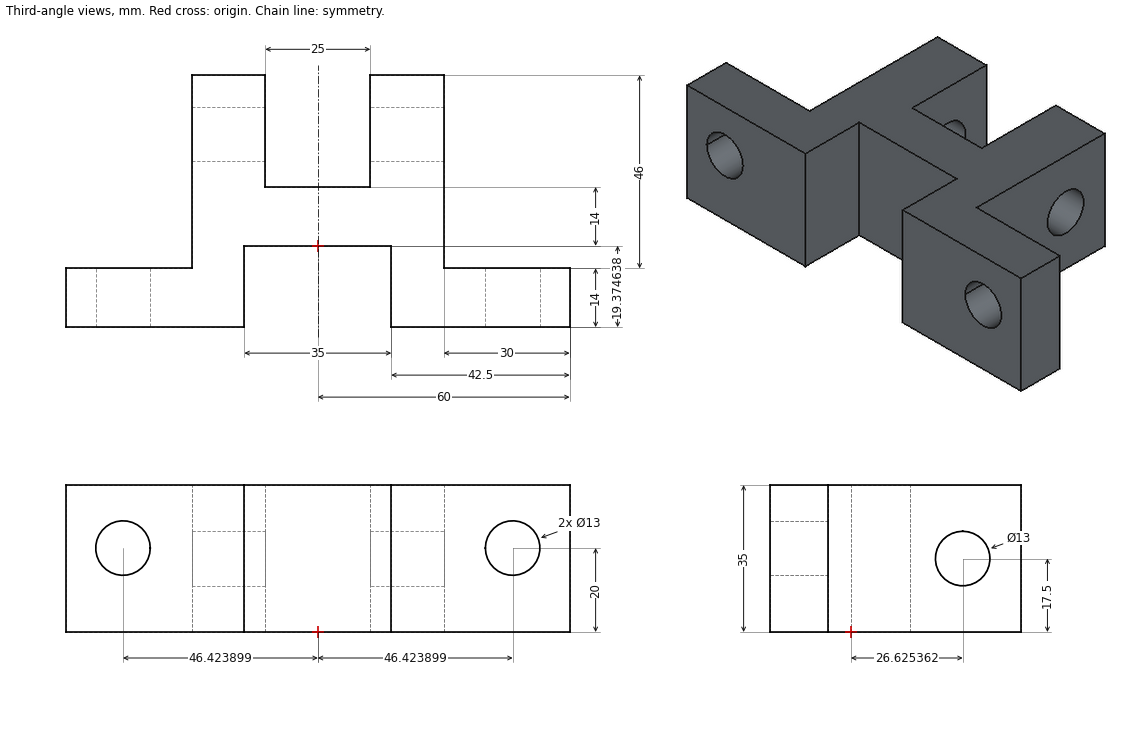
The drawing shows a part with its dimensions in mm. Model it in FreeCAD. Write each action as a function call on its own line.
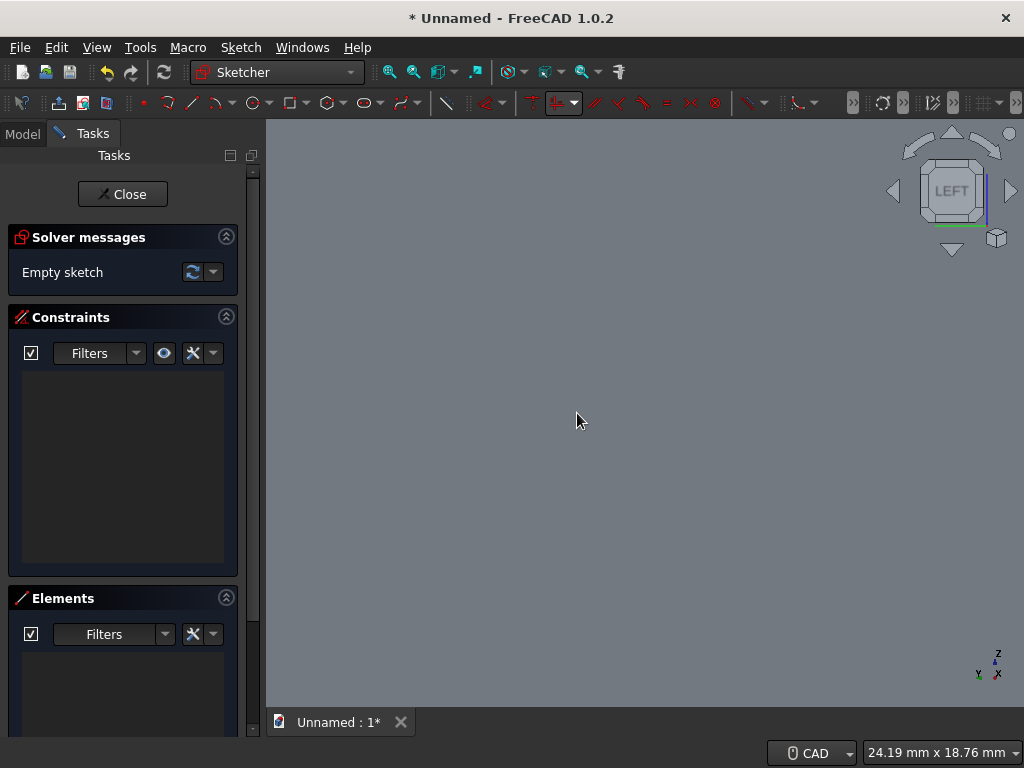
click(254, 104)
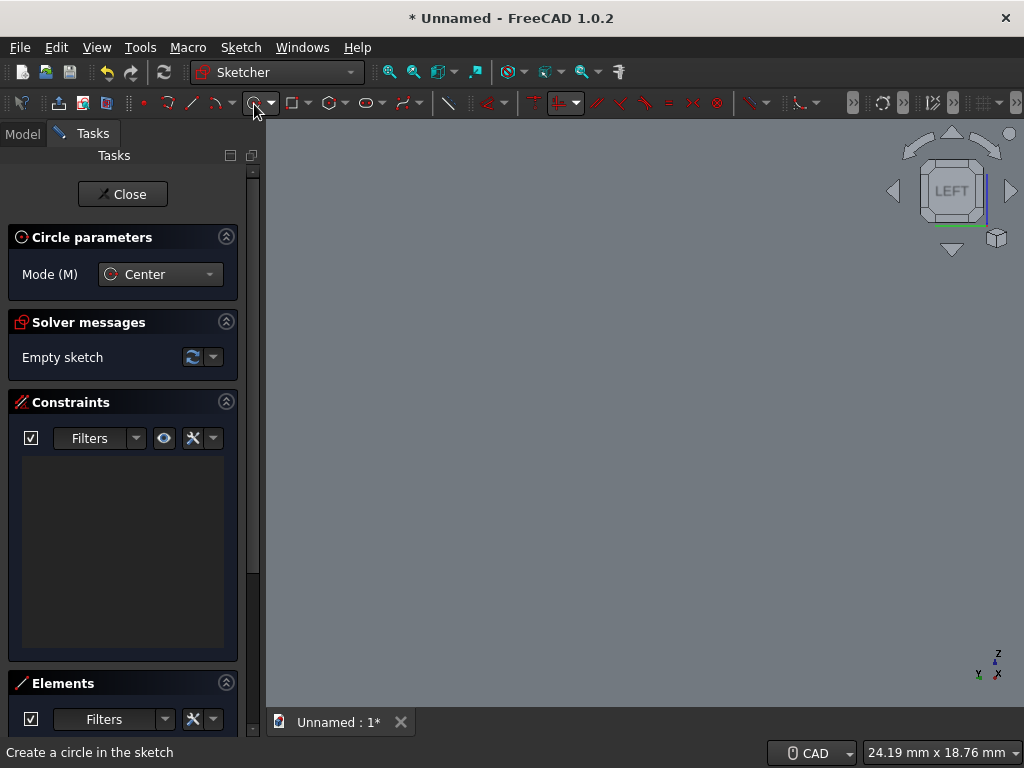
click(575, 410)
click(719, 266)
key(Escape)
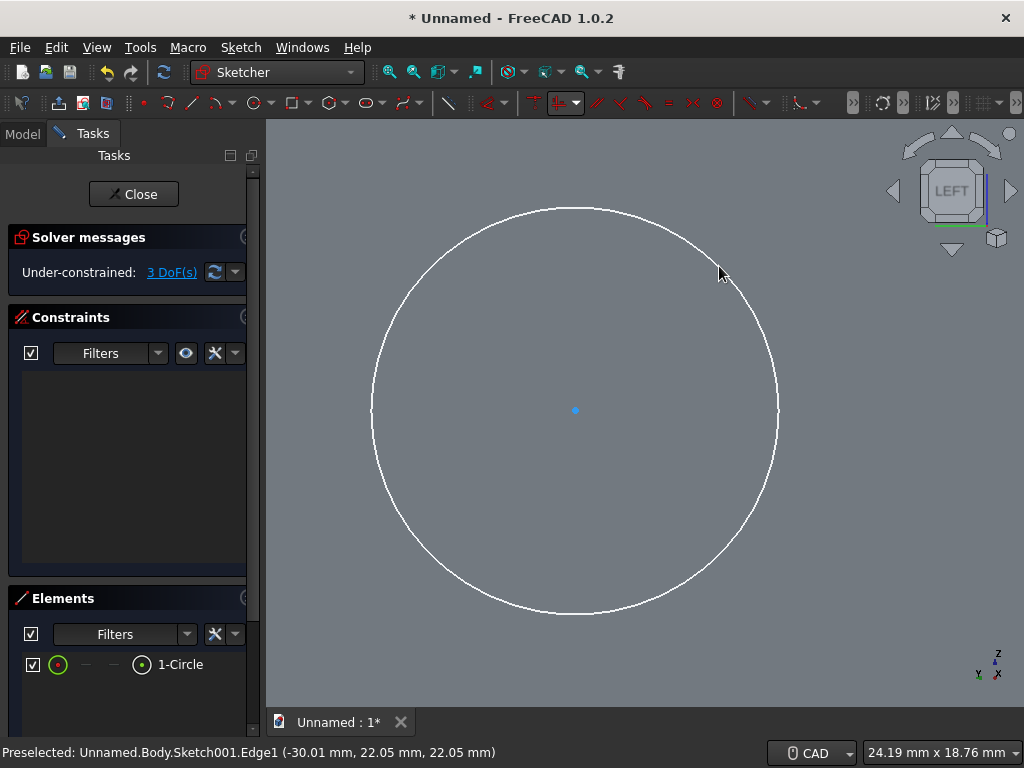
click(488, 104)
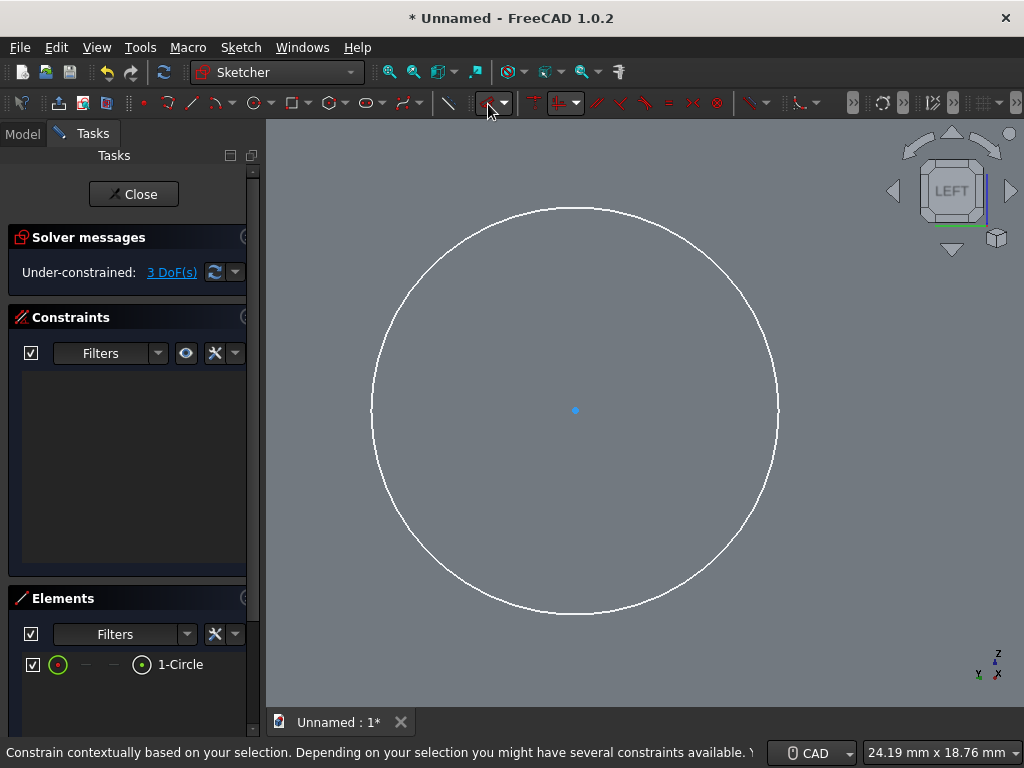
click(719, 267)
click(742, 244)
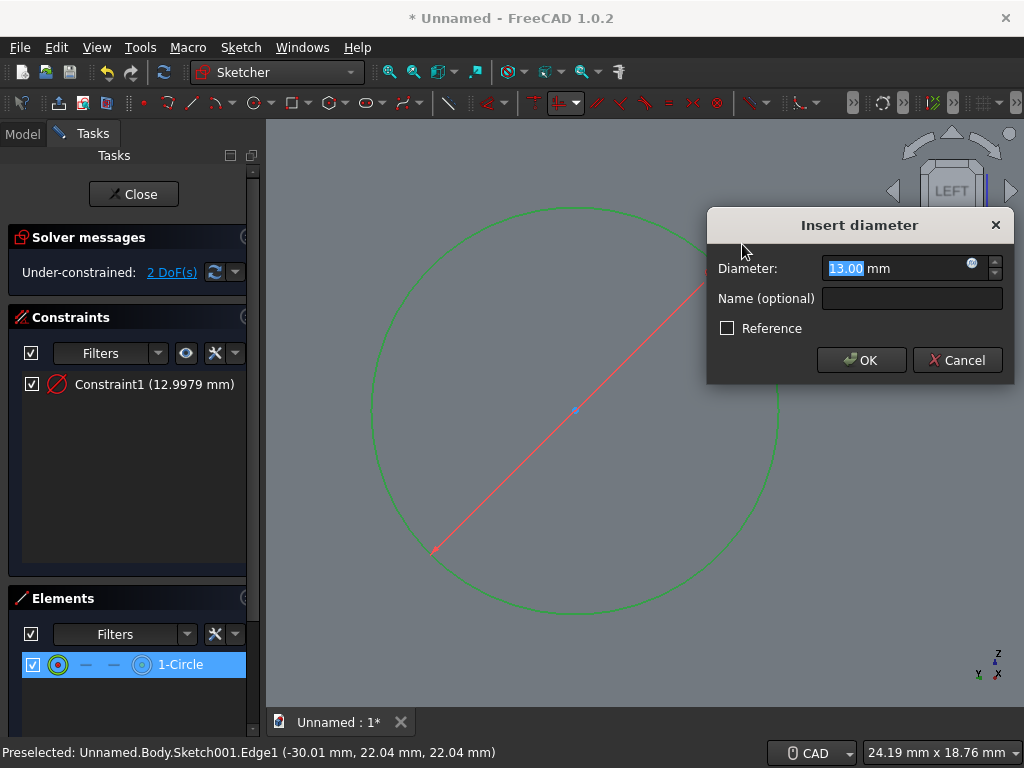
text(13)
key(Return)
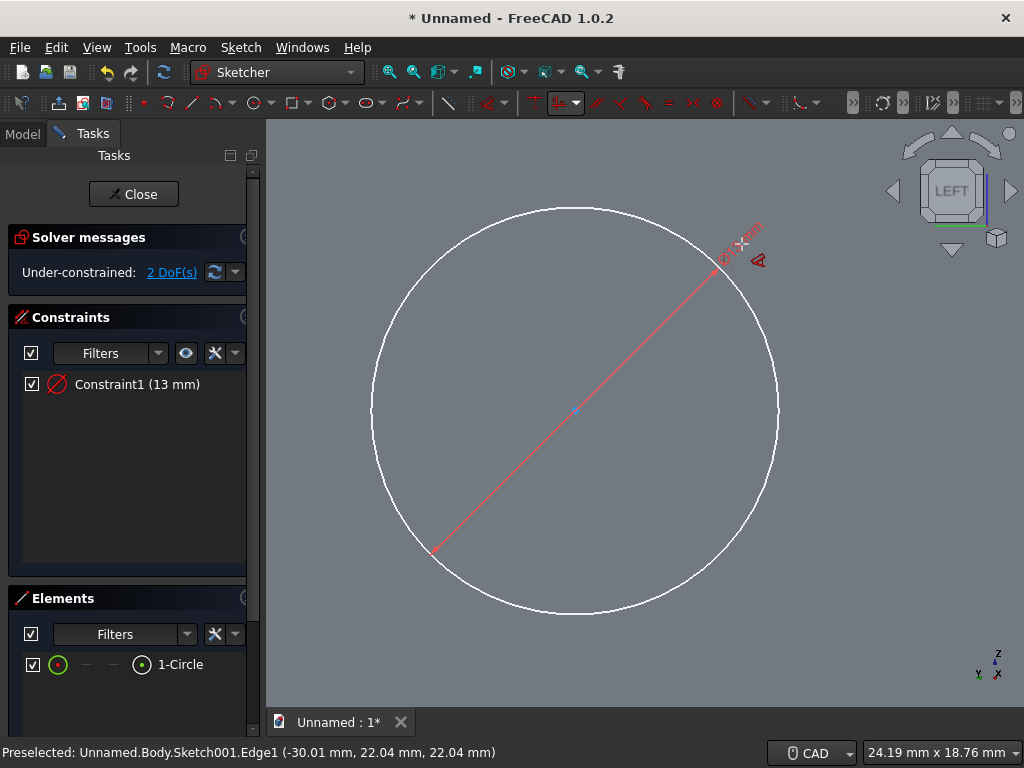
click(575, 411)
click(541, 545)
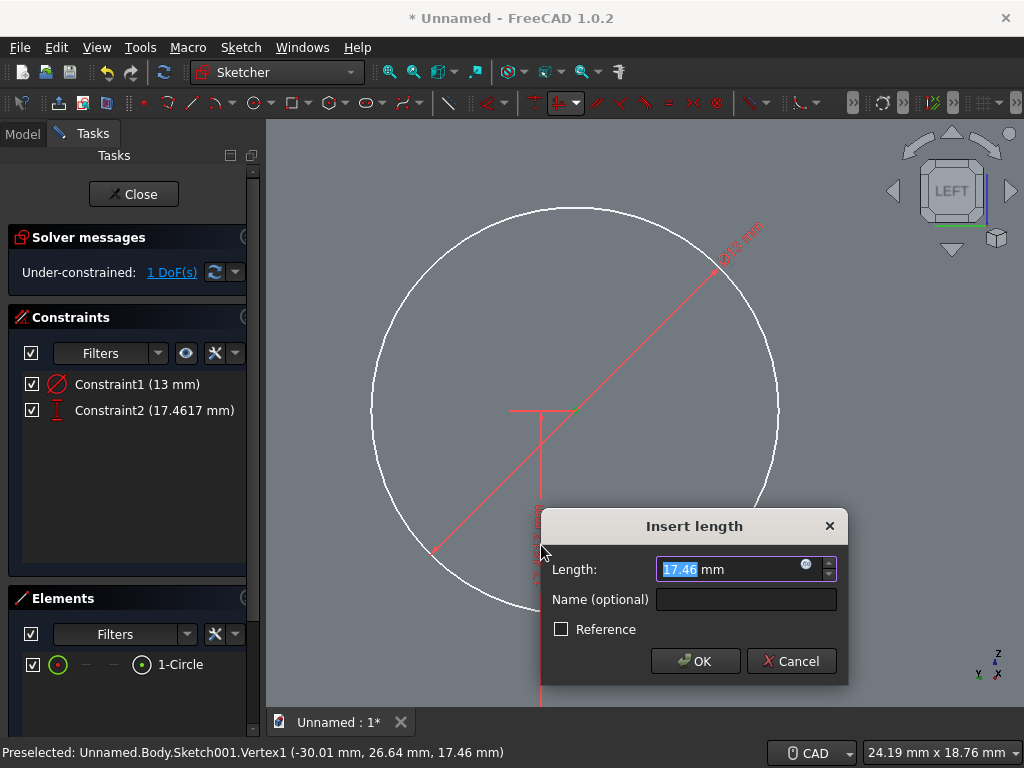
text(17.5)
key(Return)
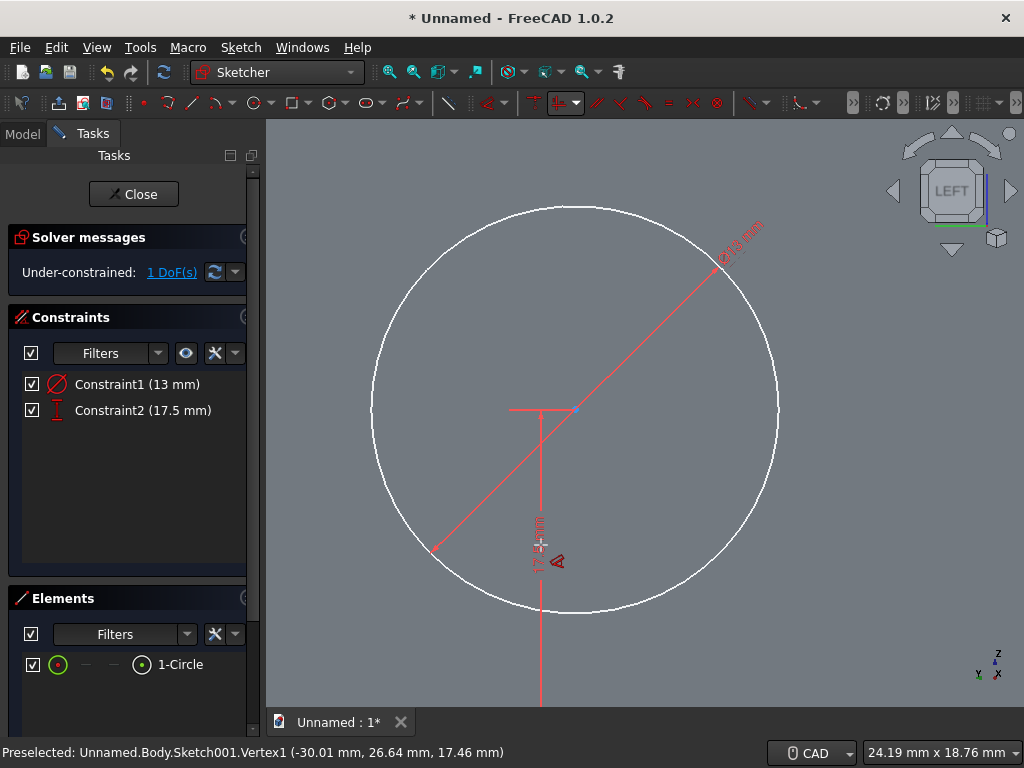
click(575, 410)
click(717, 376)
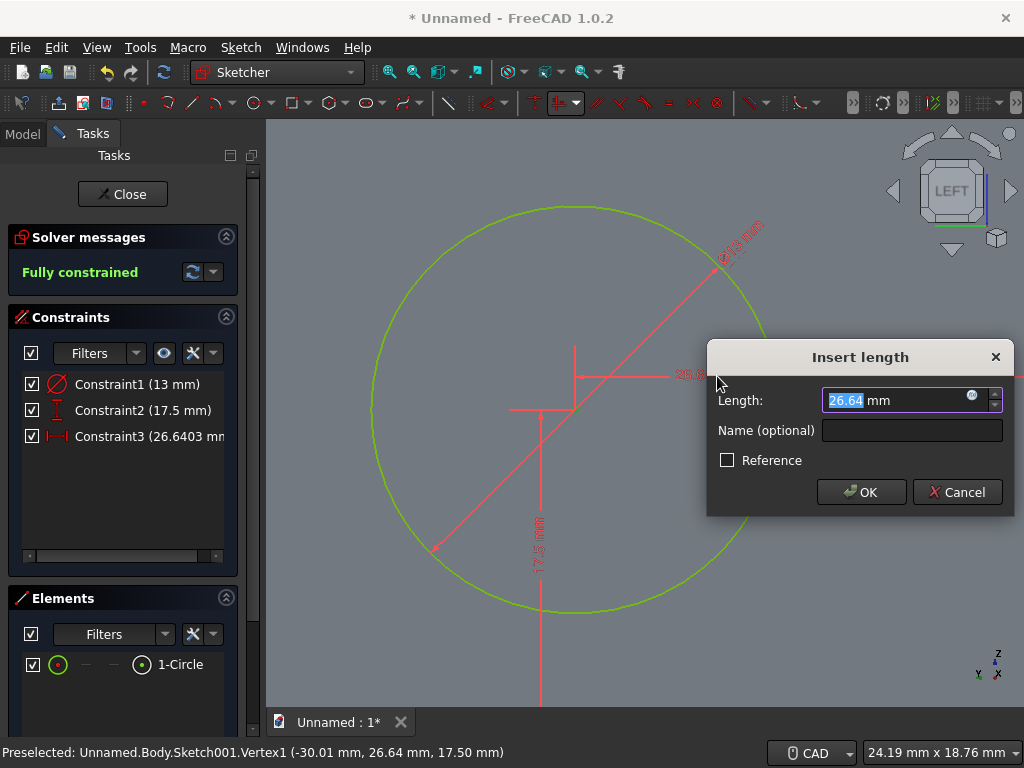
text(26.625362)
key(Return)
key(Escape)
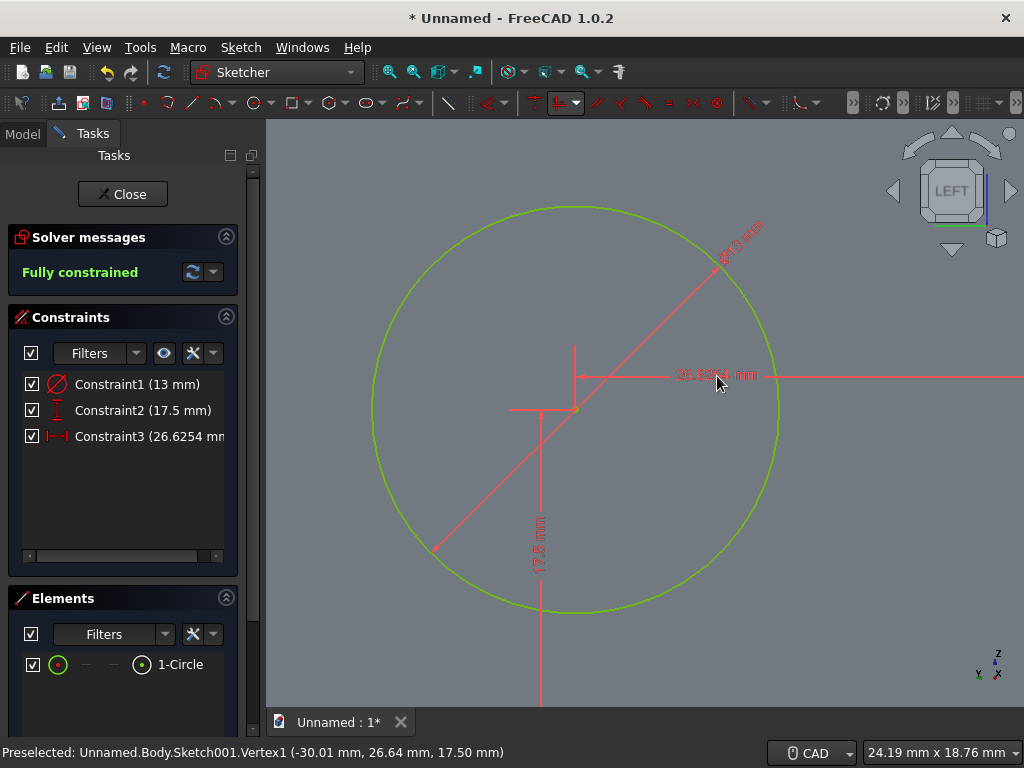
click(123, 194)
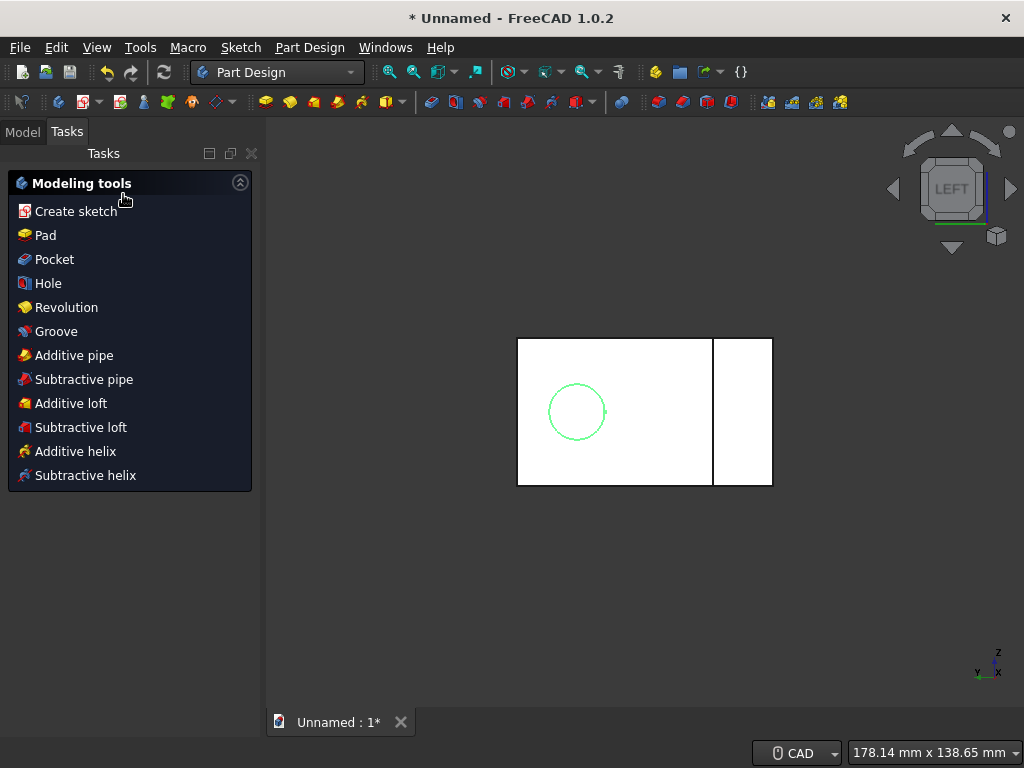
click(432, 102)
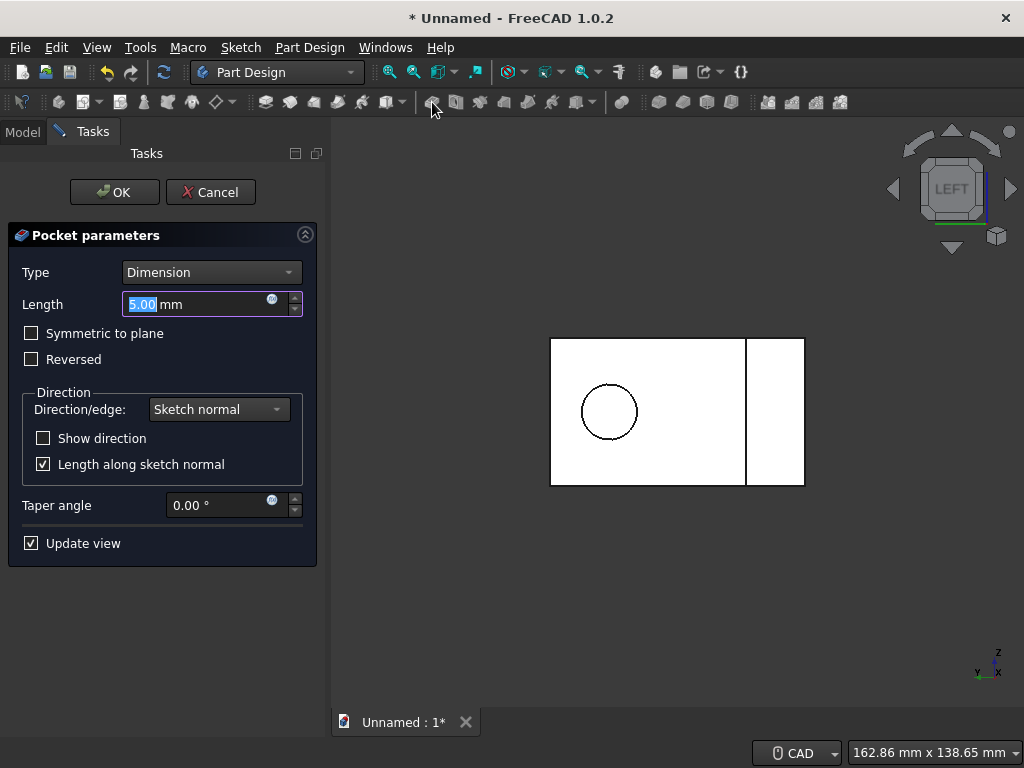
click(212, 272)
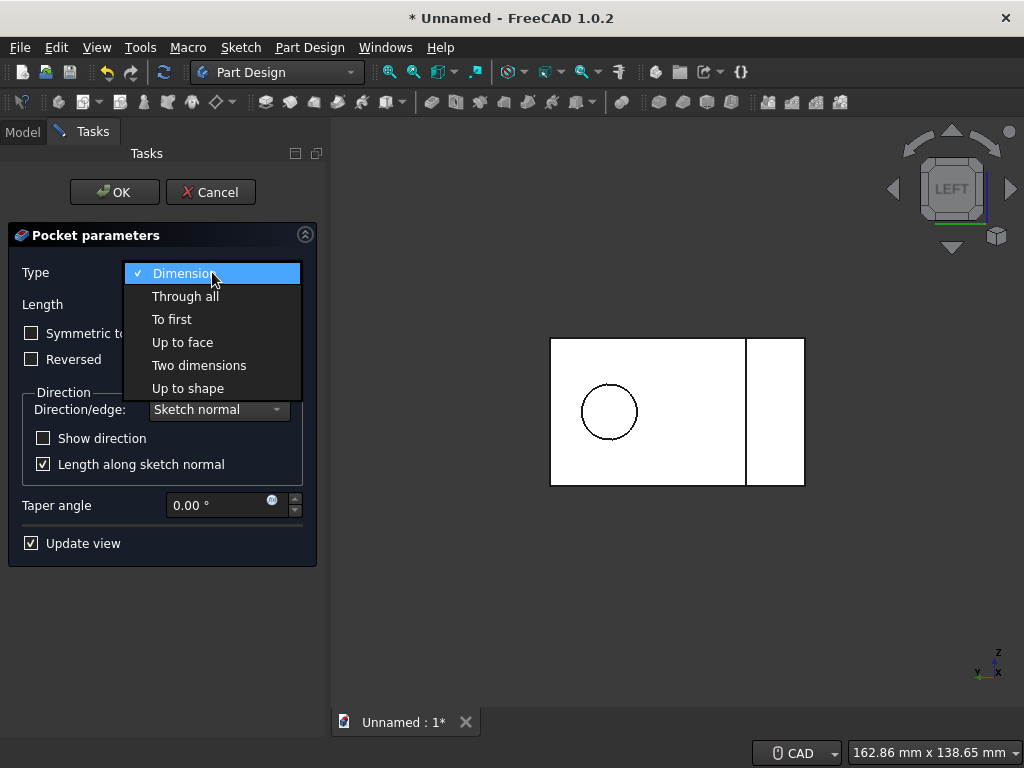
click(212, 296)